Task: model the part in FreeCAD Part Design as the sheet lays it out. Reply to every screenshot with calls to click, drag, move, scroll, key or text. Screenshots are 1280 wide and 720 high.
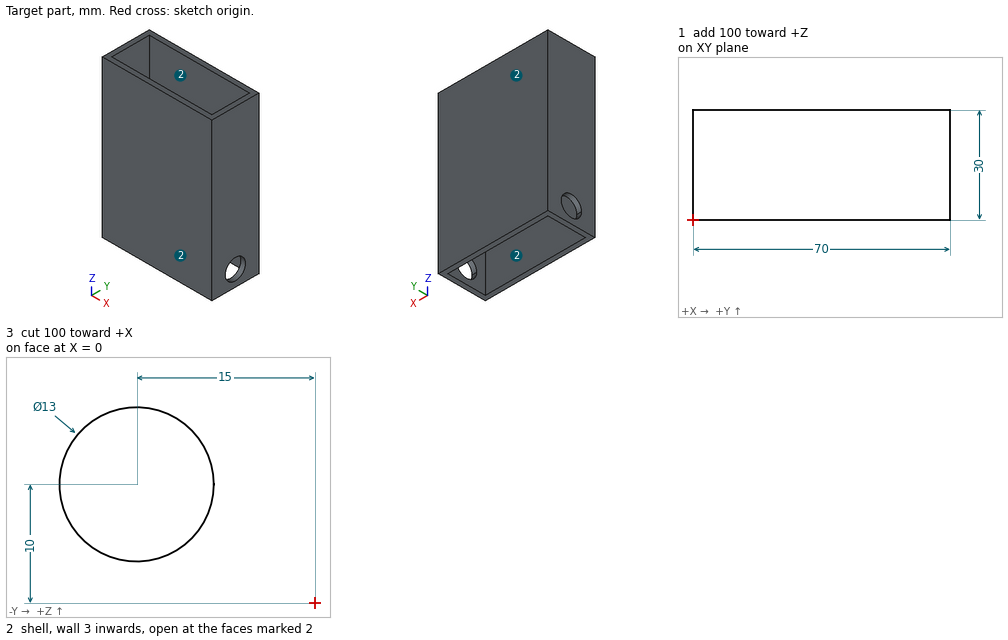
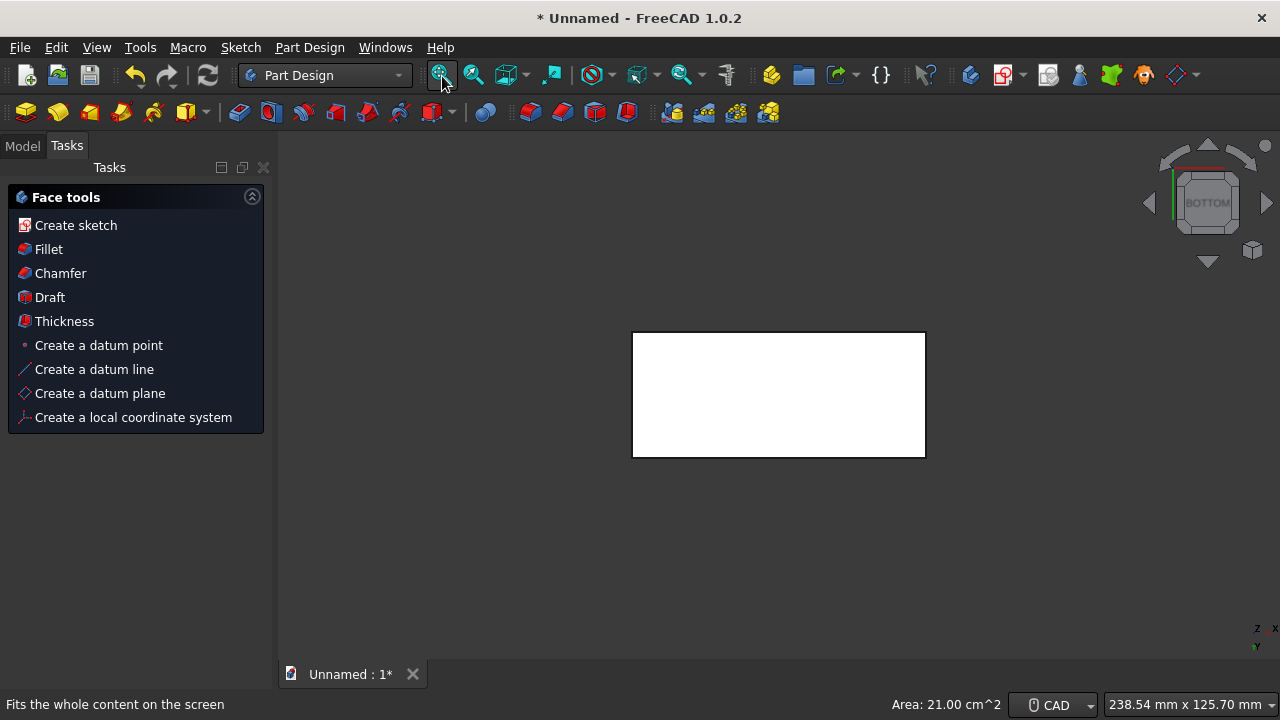
click(863, 394, ctrl)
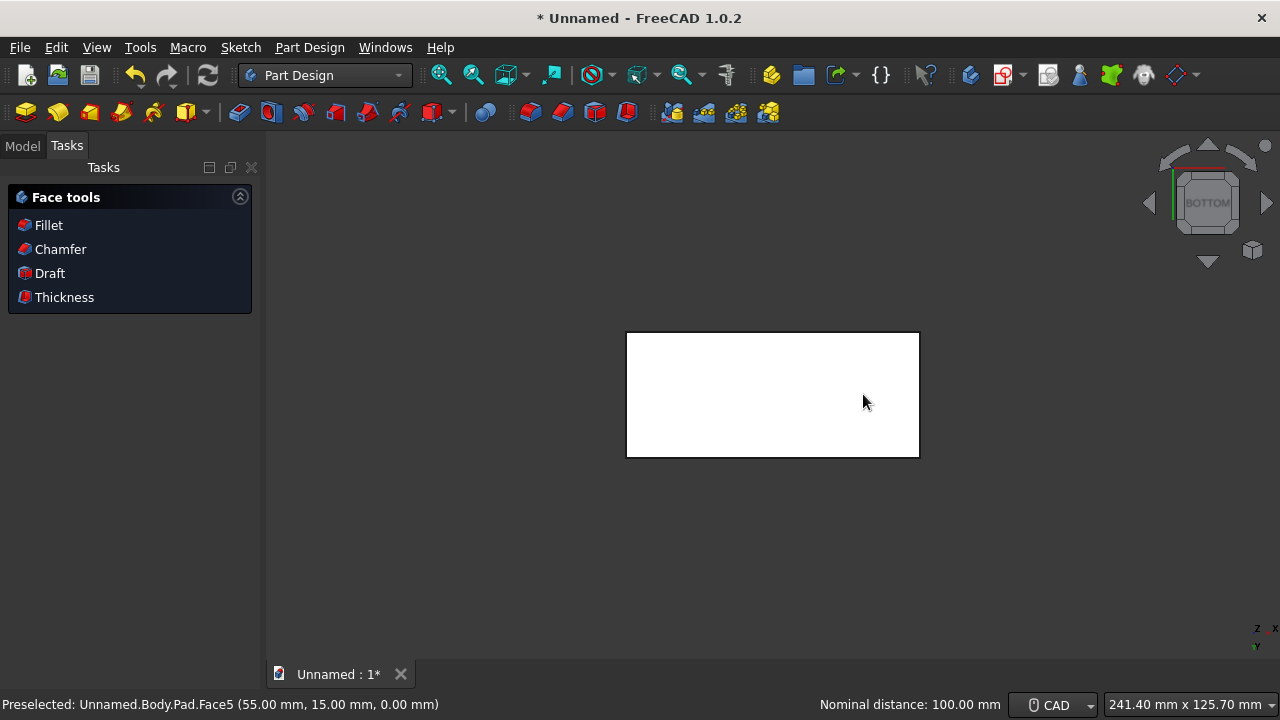
click(628, 112)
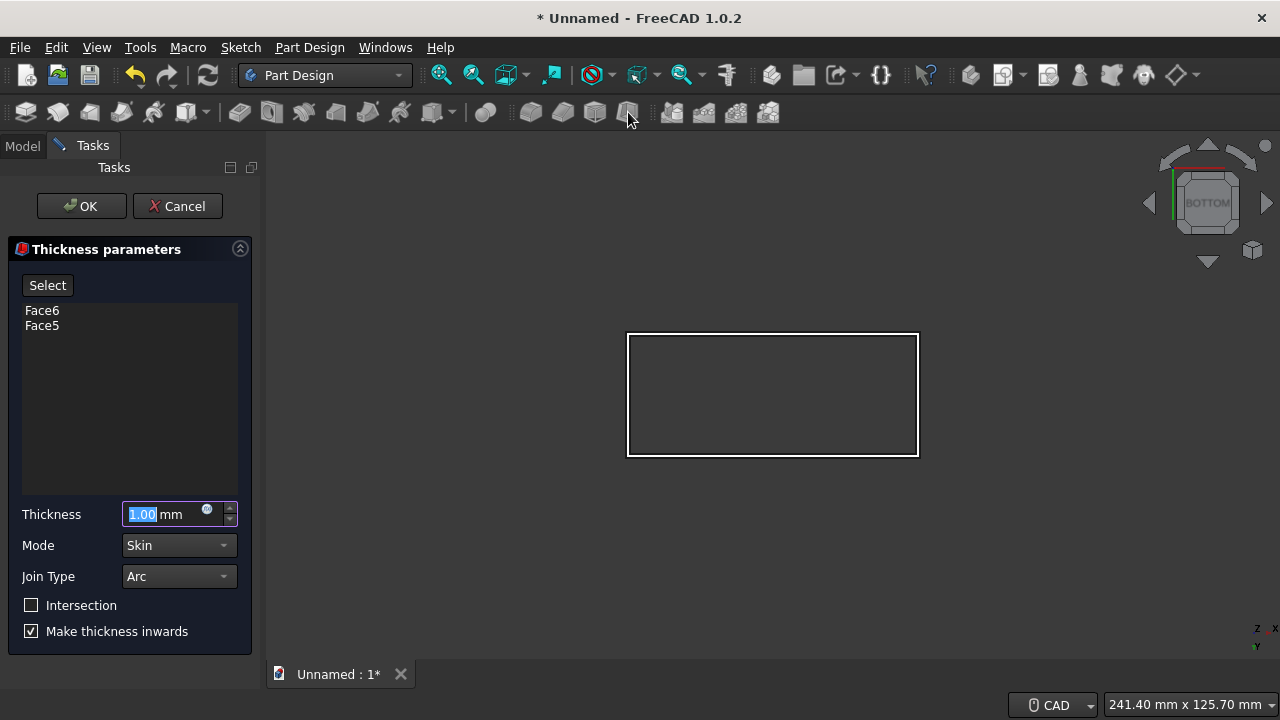
text(3)
key(Tab)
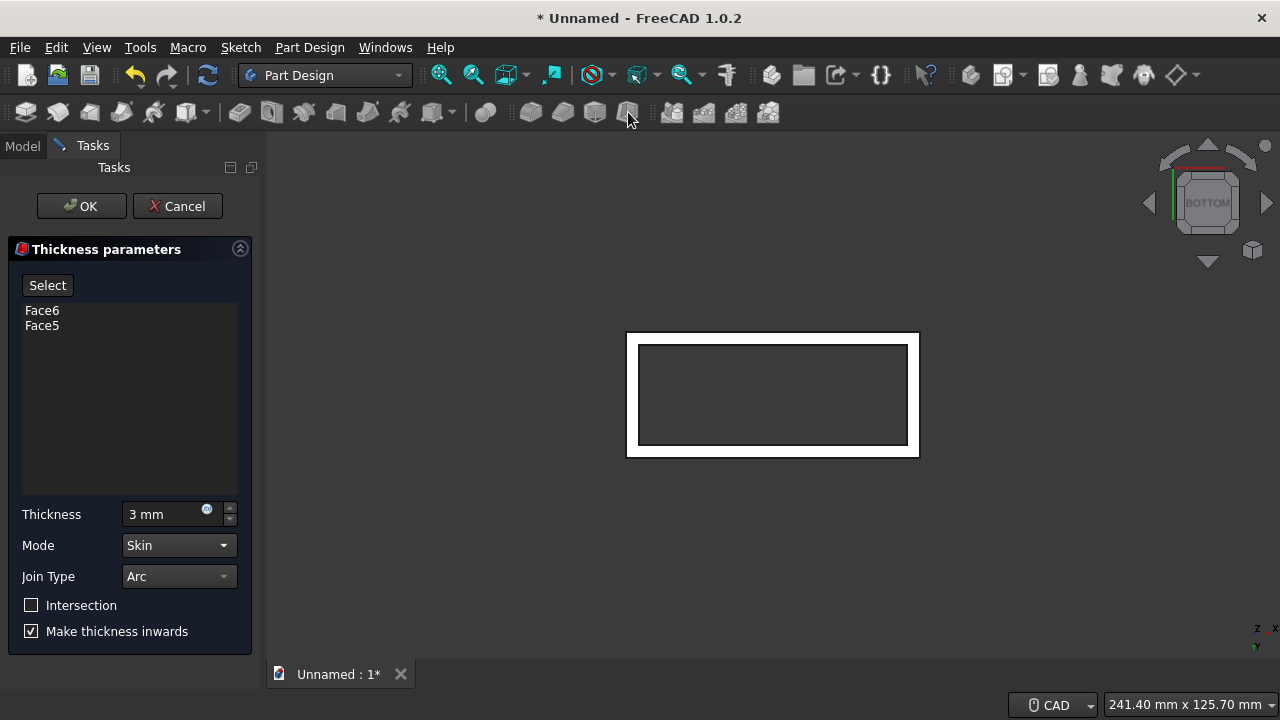
click(180, 576)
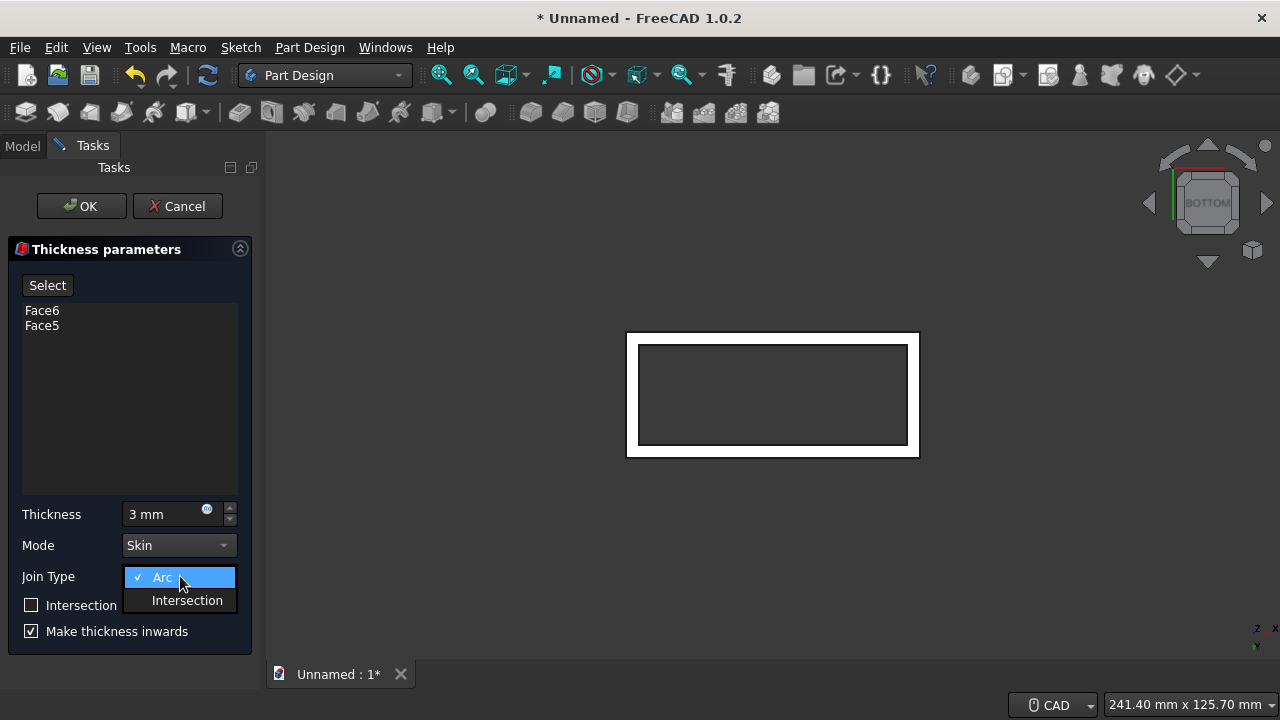
click(179, 600)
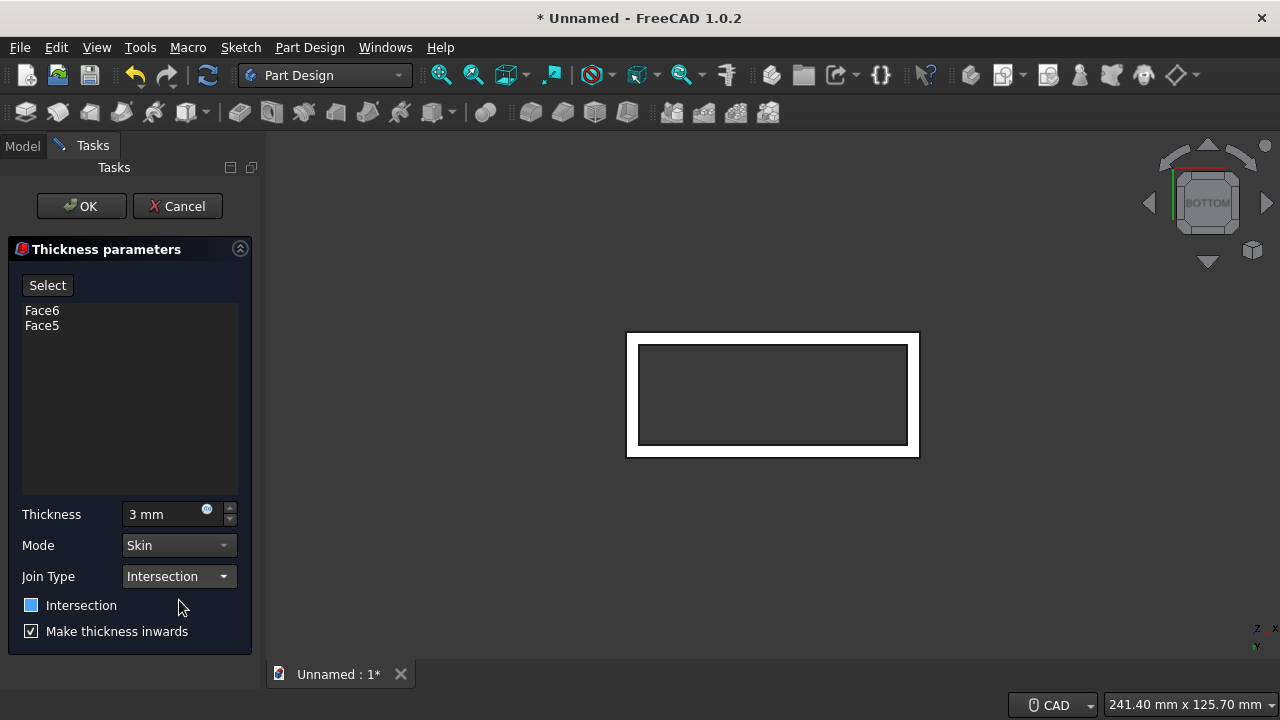
click(82, 206)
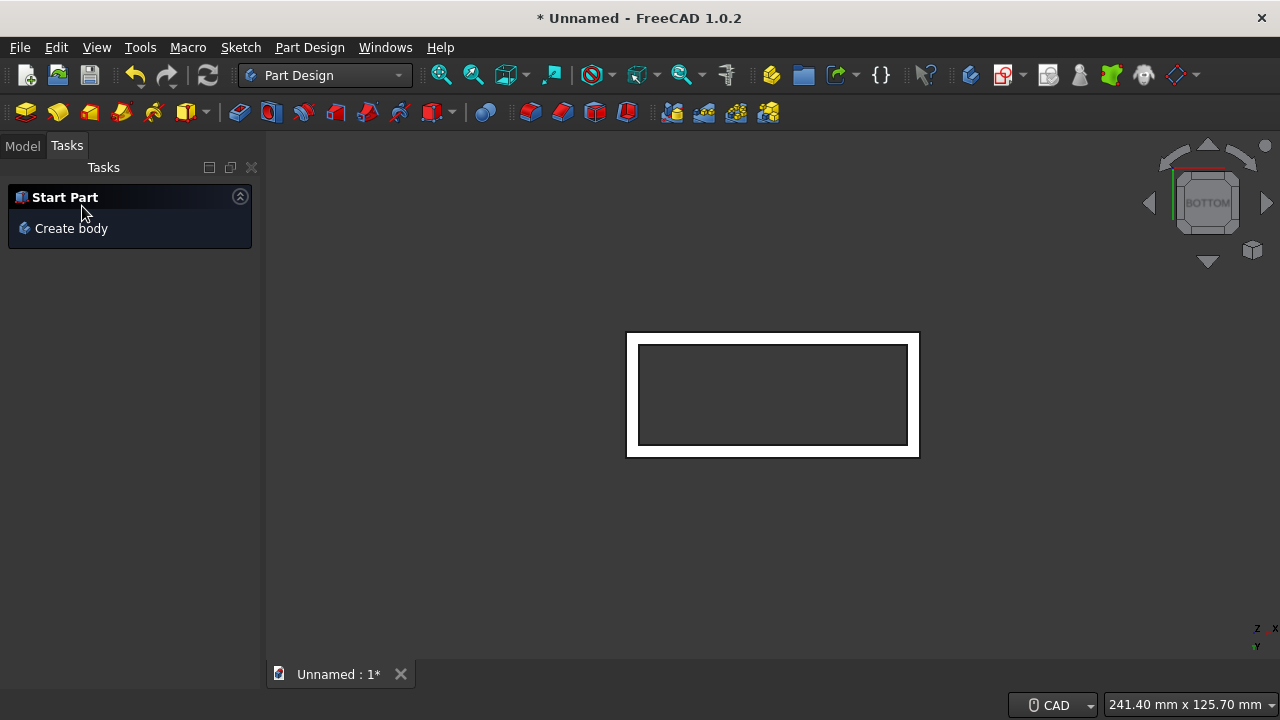
key(v)
key(f)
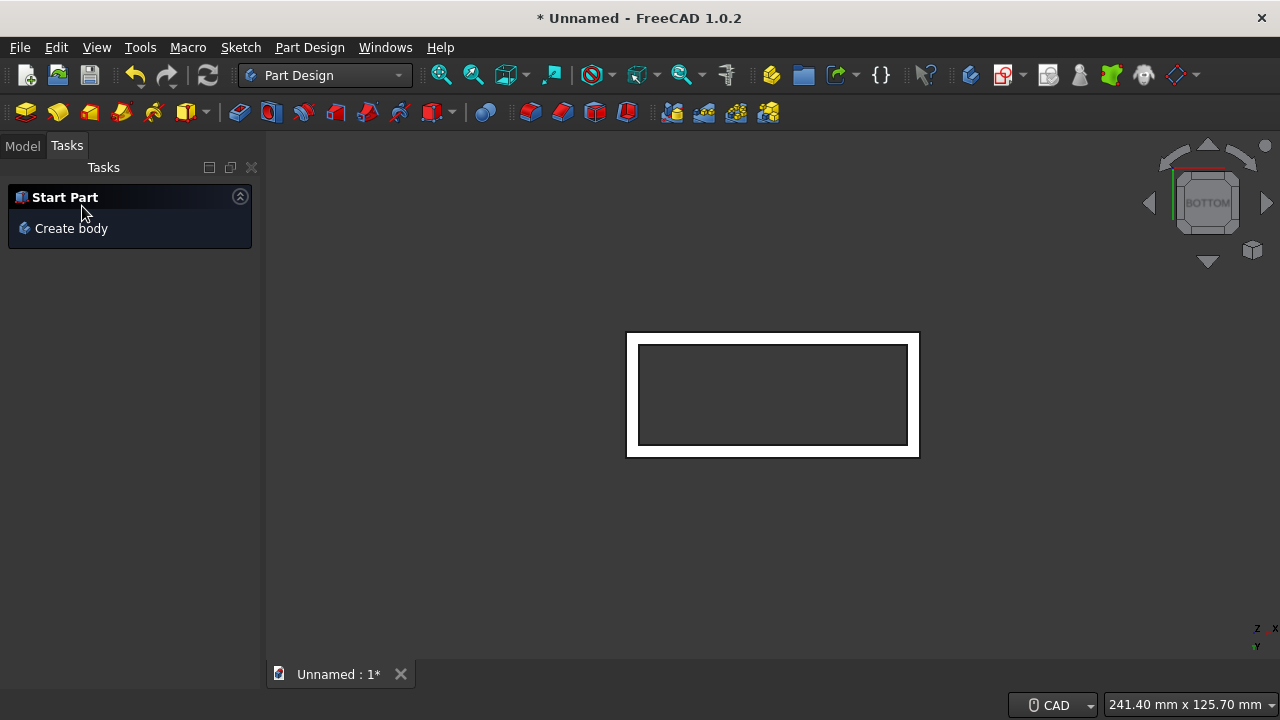
key(6)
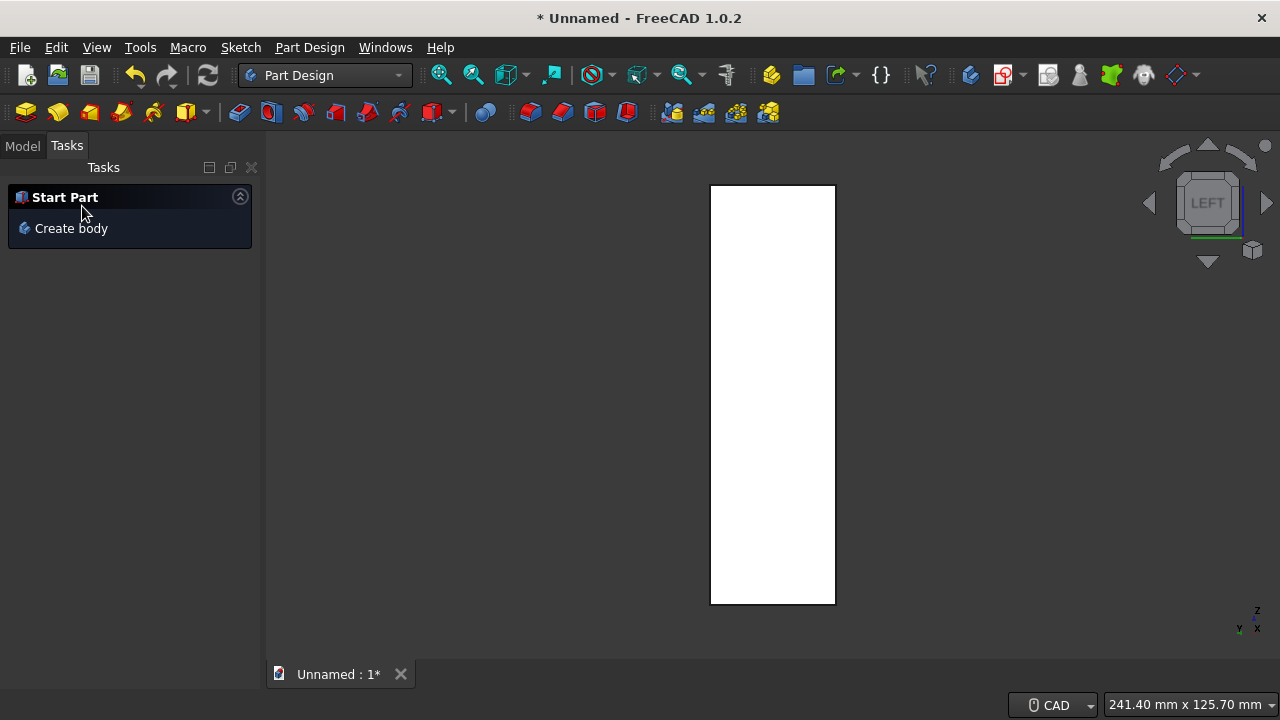
click(773, 274)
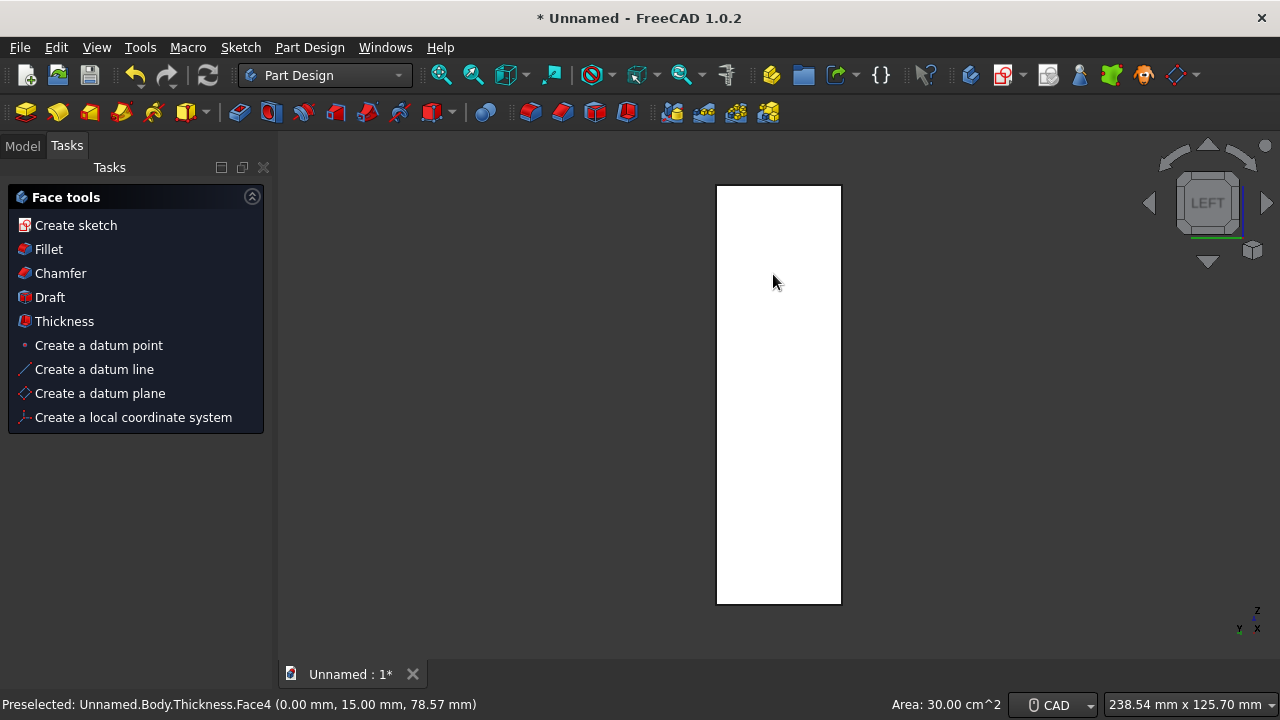
click(1004, 76)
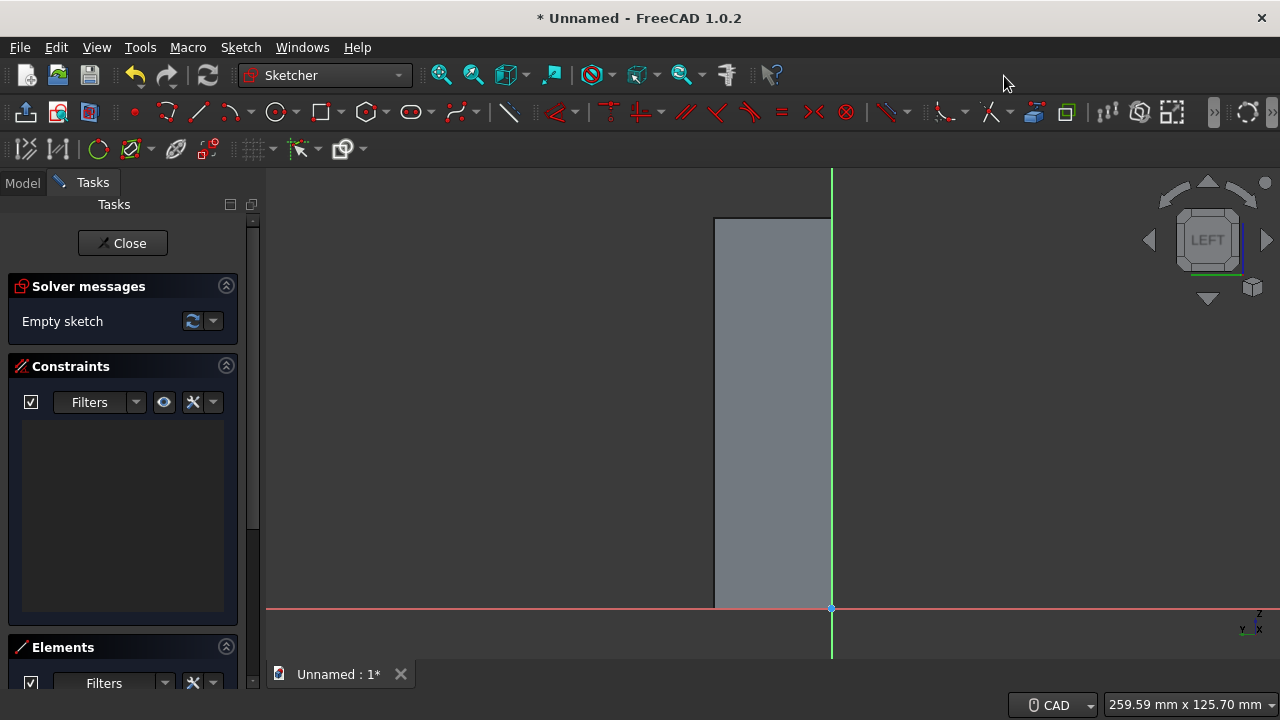
scroll(811, 618, up, 8)